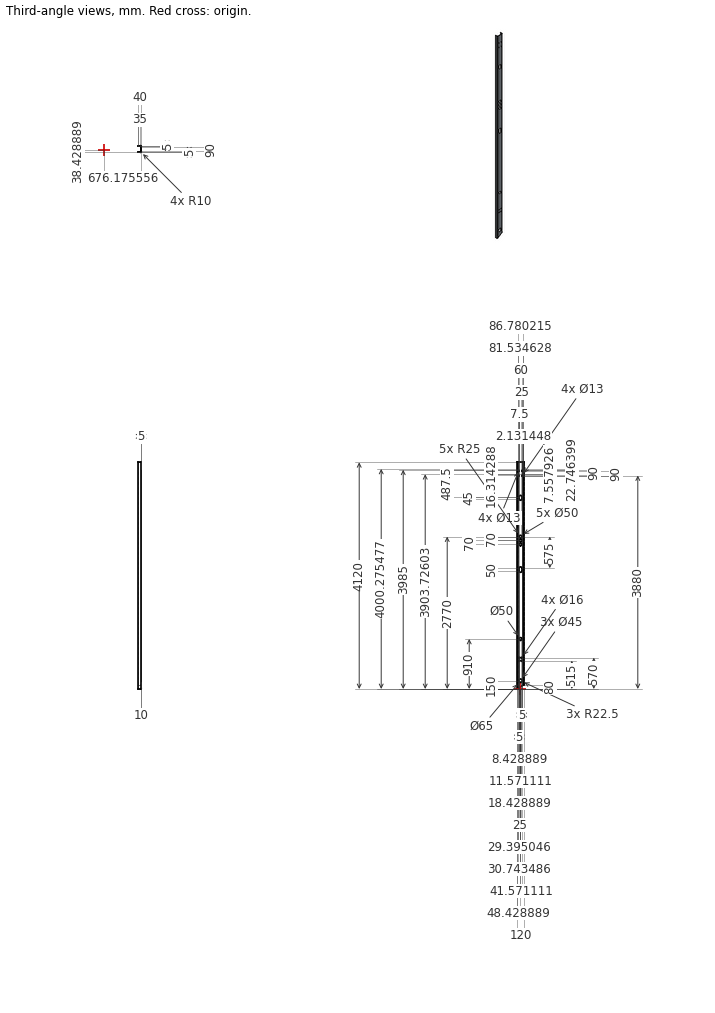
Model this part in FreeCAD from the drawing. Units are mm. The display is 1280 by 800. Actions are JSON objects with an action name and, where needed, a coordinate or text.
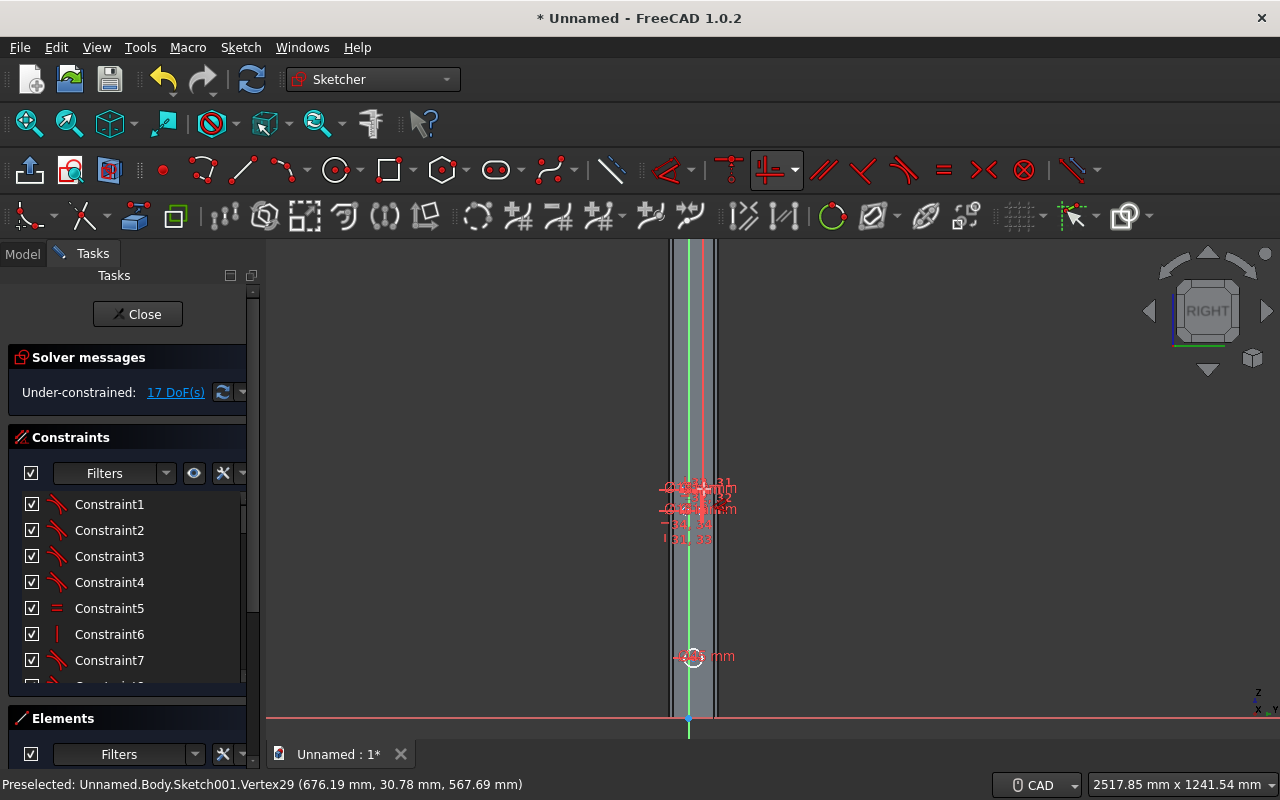
{"action": "scroll", "coordinate": [707, 634], "scroll_direction": "down", "scroll_amount": 8}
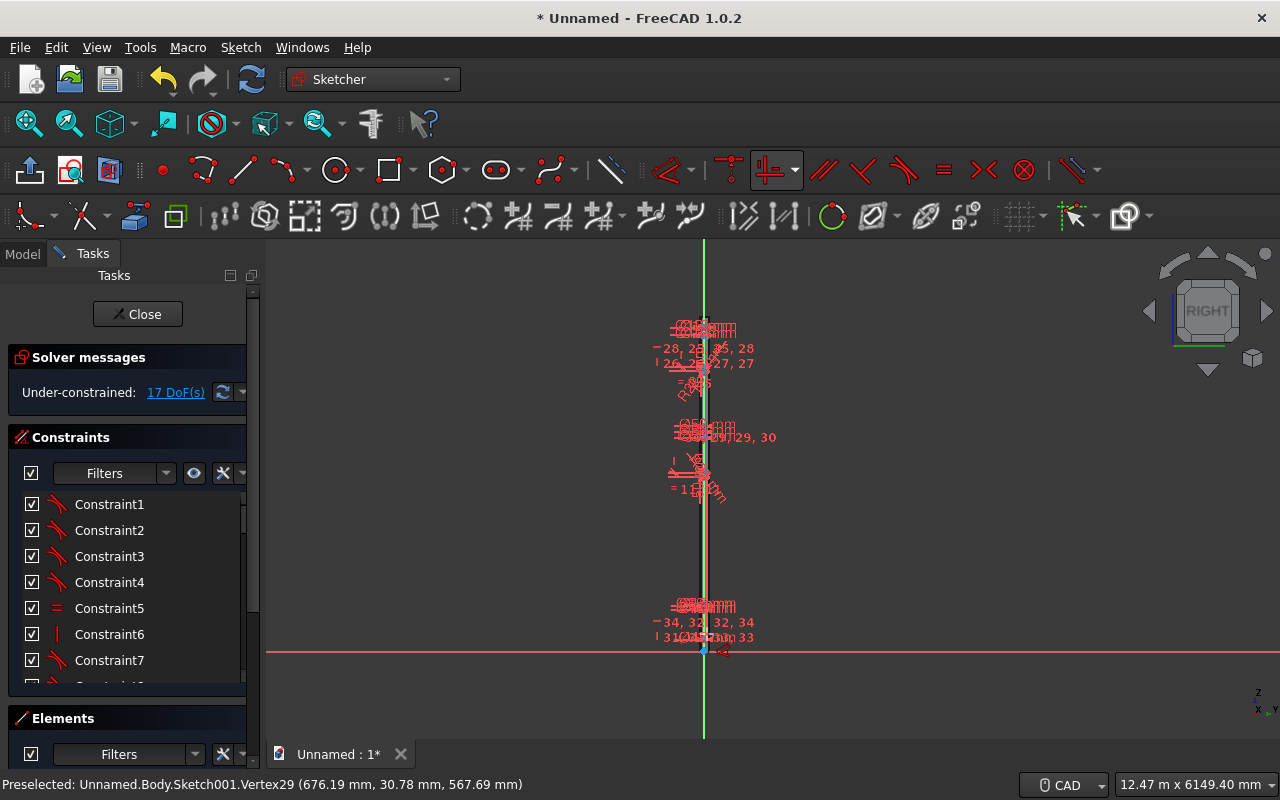
{"action": "scroll", "coordinate": [703, 477], "scroll_direction": "up", "scroll_amount": 23}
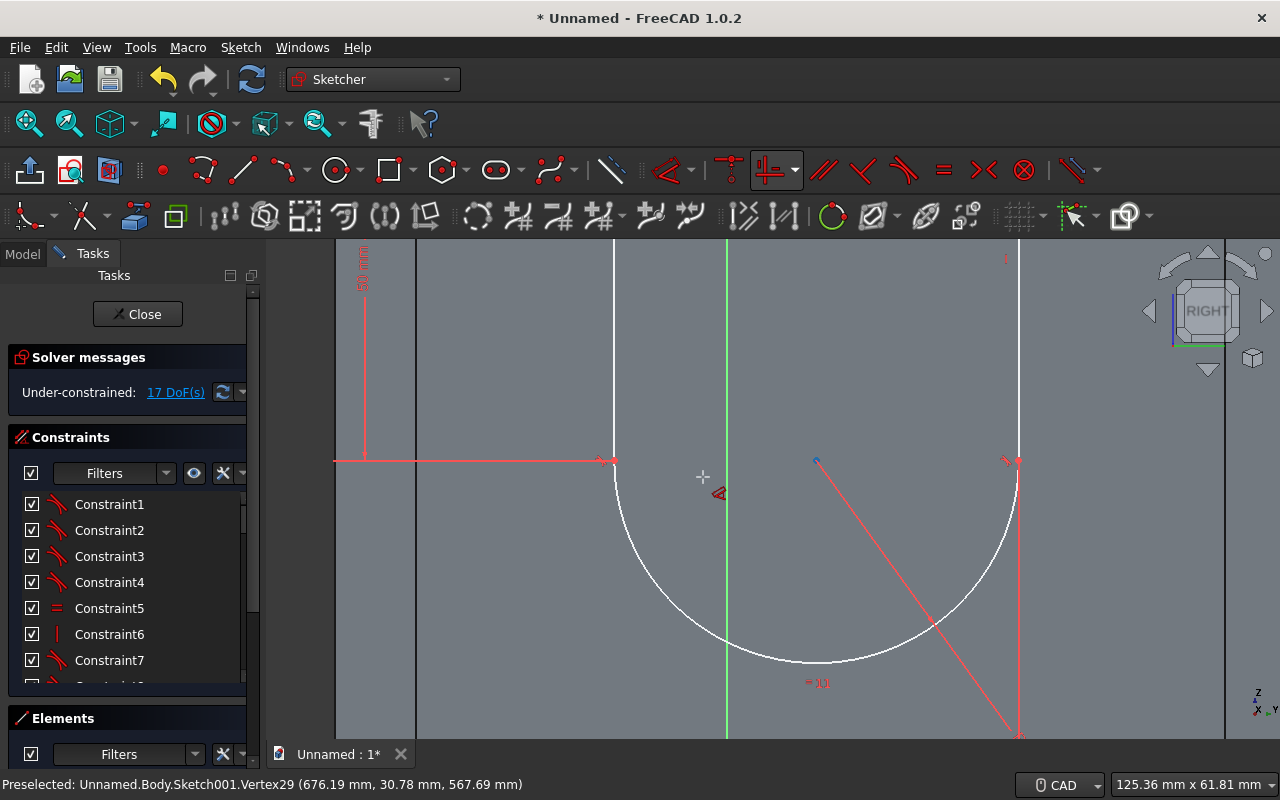
{"action": "left_click", "coordinate": [614, 461]}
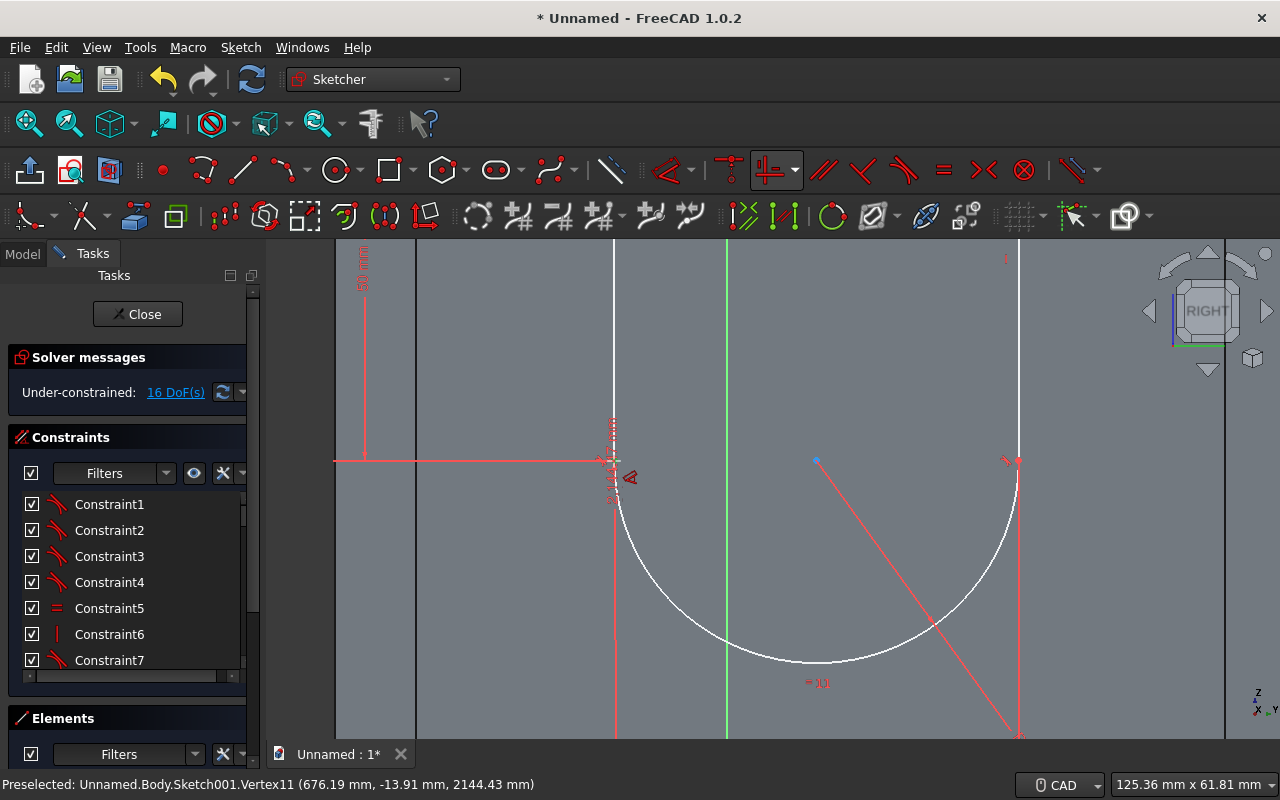
{"action": "scroll", "coordinate": [704, 489], "scroll_direction": "down", "scroll_amount": 15}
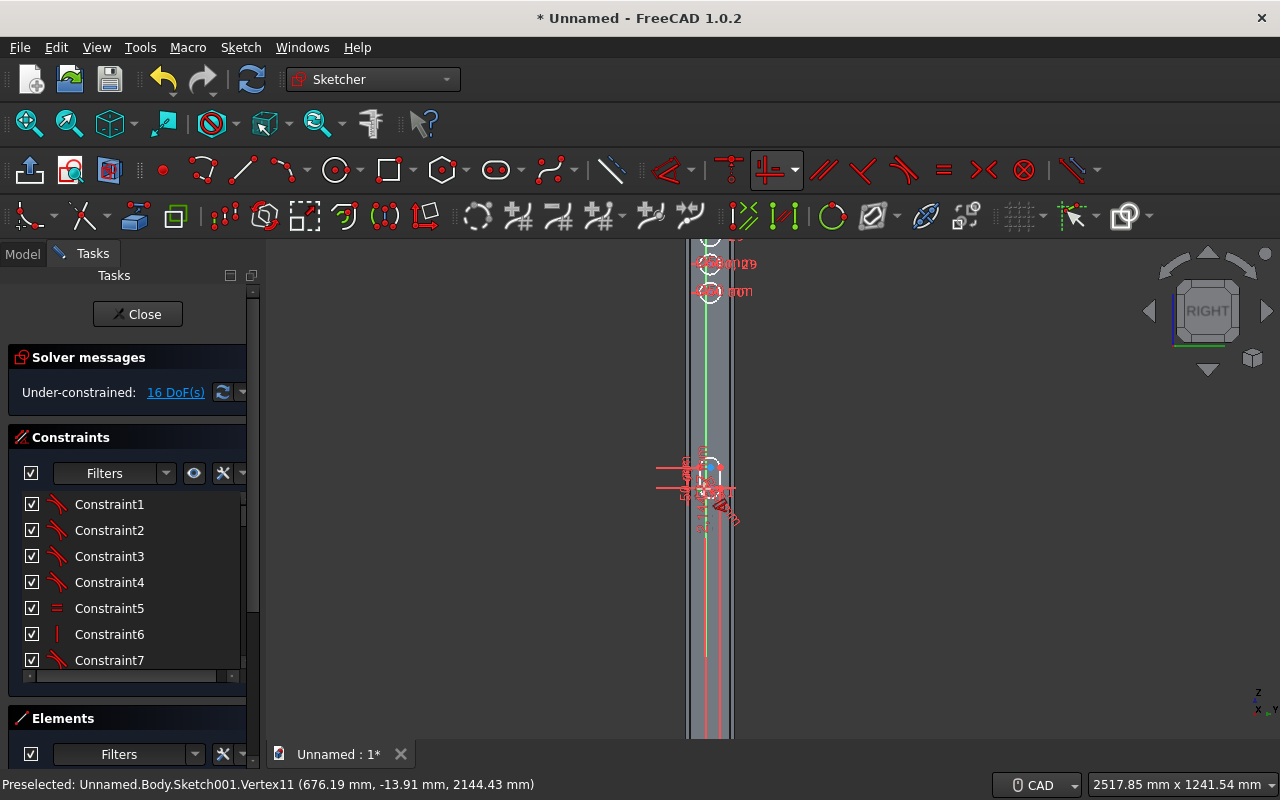
{"action": "scroll", "coordinate": [703, 474], "scroll_direction": "down", "scroll_amount": 8}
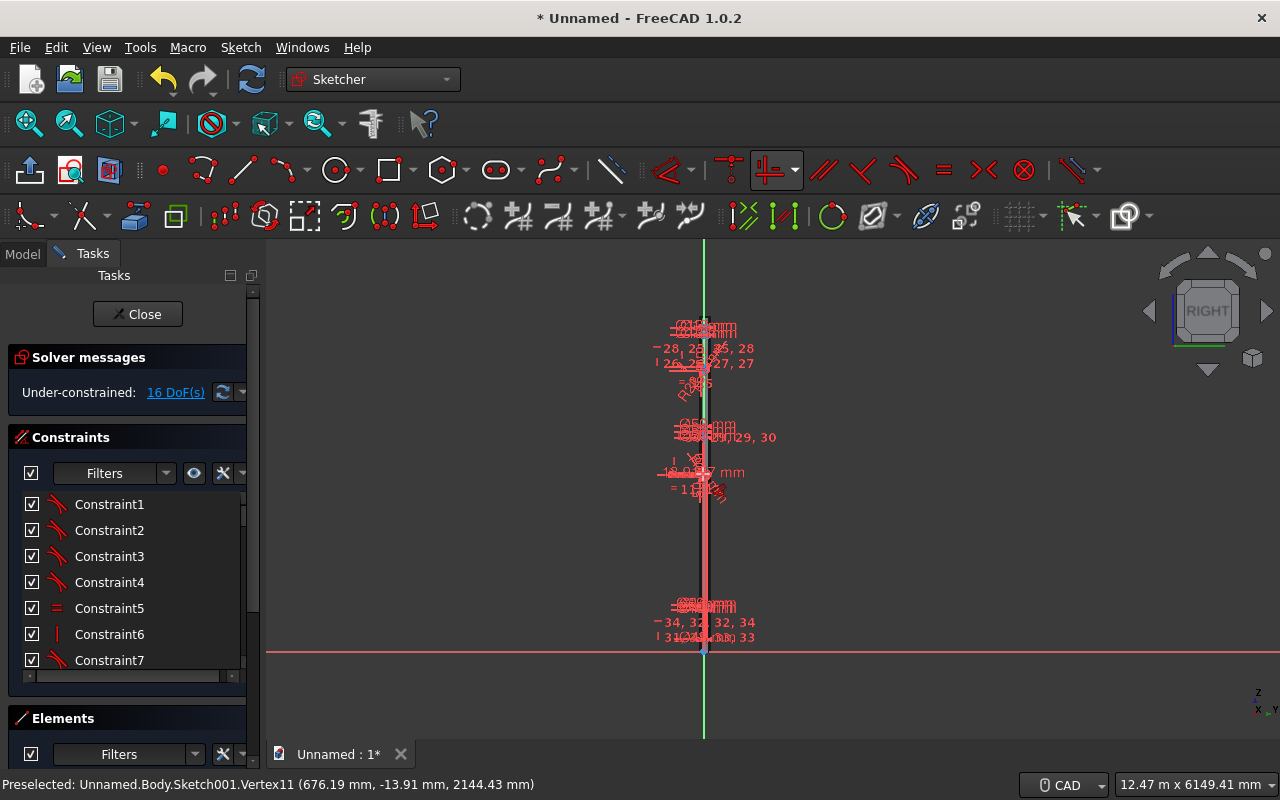
{"action": "scroll", "coordinate": [703, 605], "scroll_direction": "up", "scroll_amount": 23}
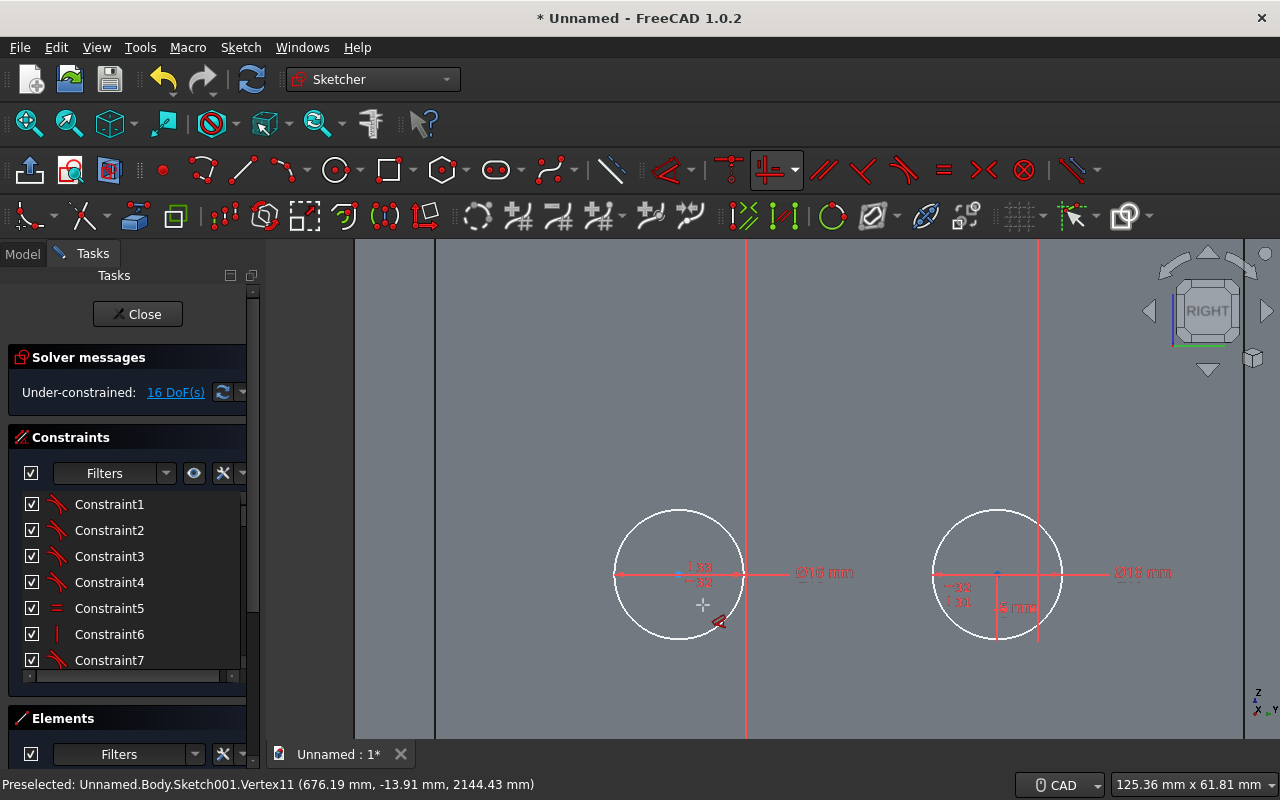
{"action": "left_click", "coordinate": [679, 575]}
{"action": "left_click", "coordinate": [656, 609]}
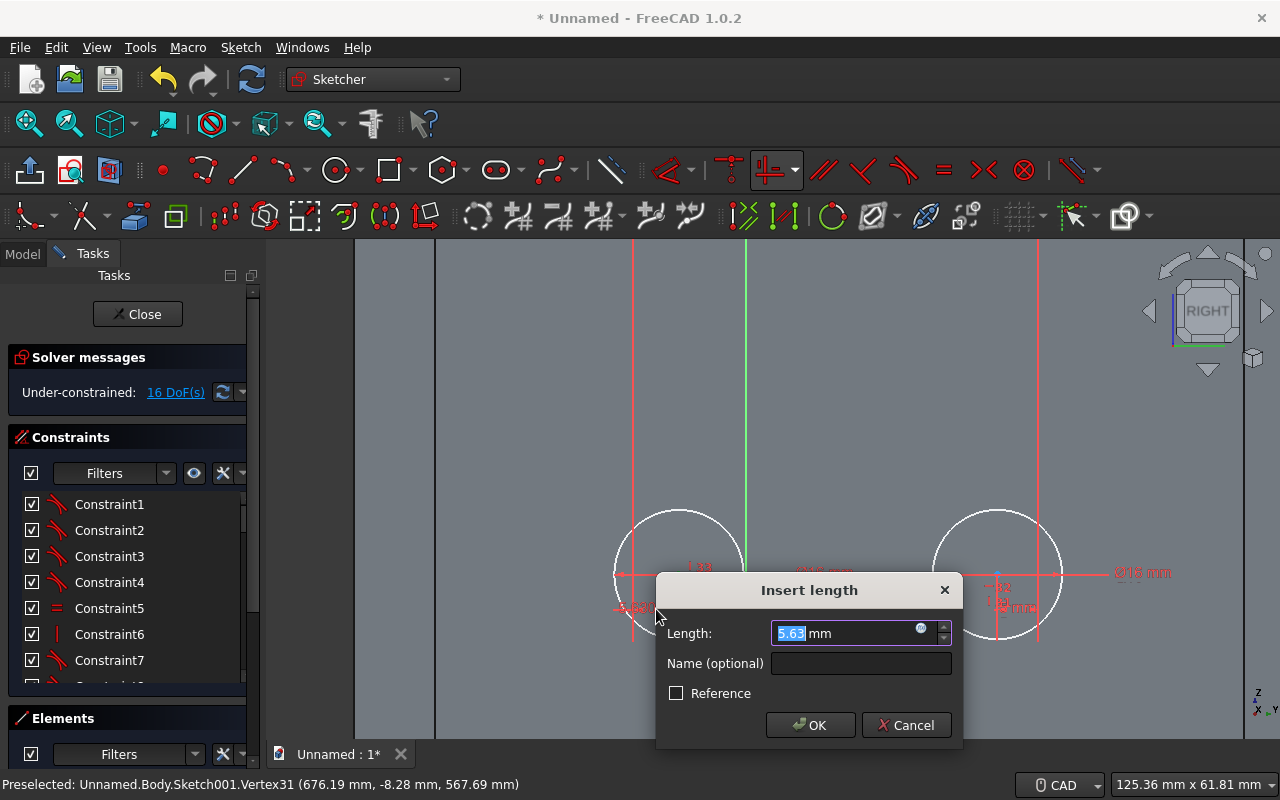
{"action": "type", "text": "5"}
{"action": "key", "text": "Return"}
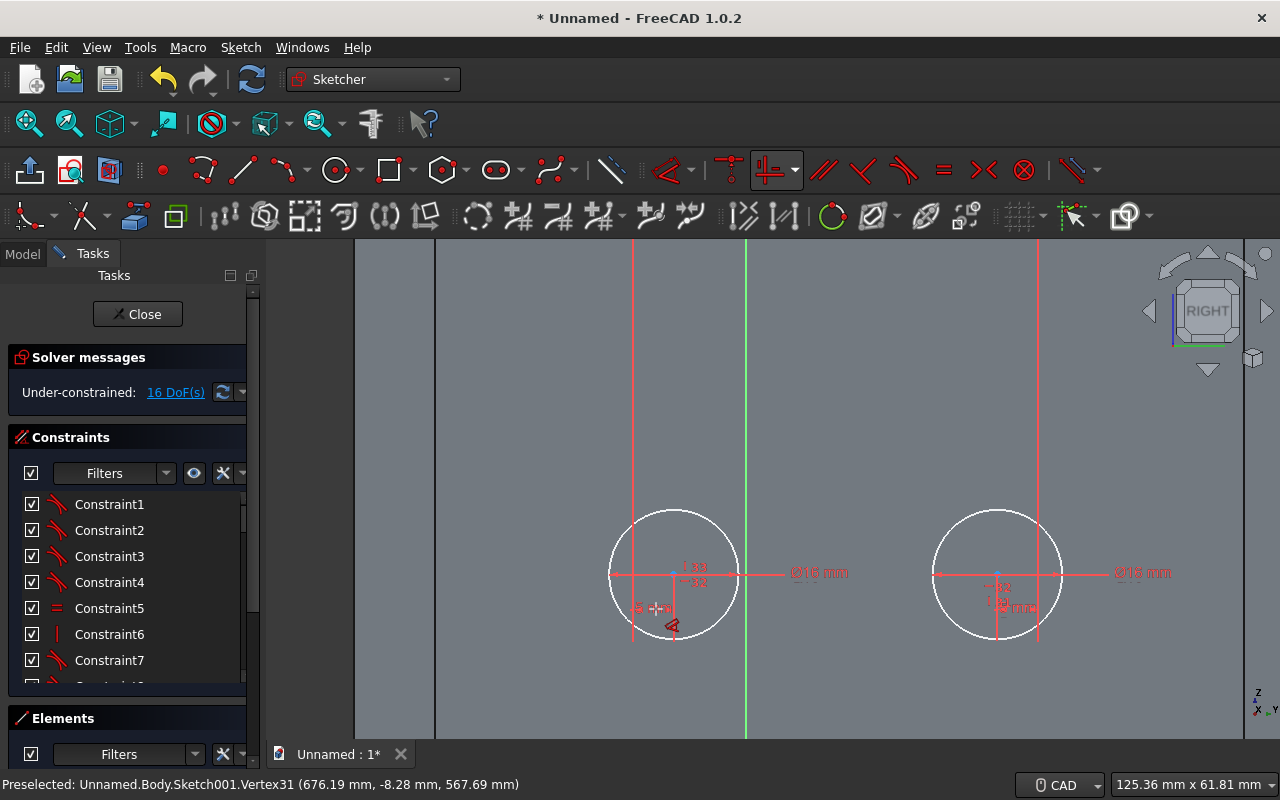
{"action": "scroll", "coordinate": [704, 489], "scroll_direction": "down", "scroll_amount": 15}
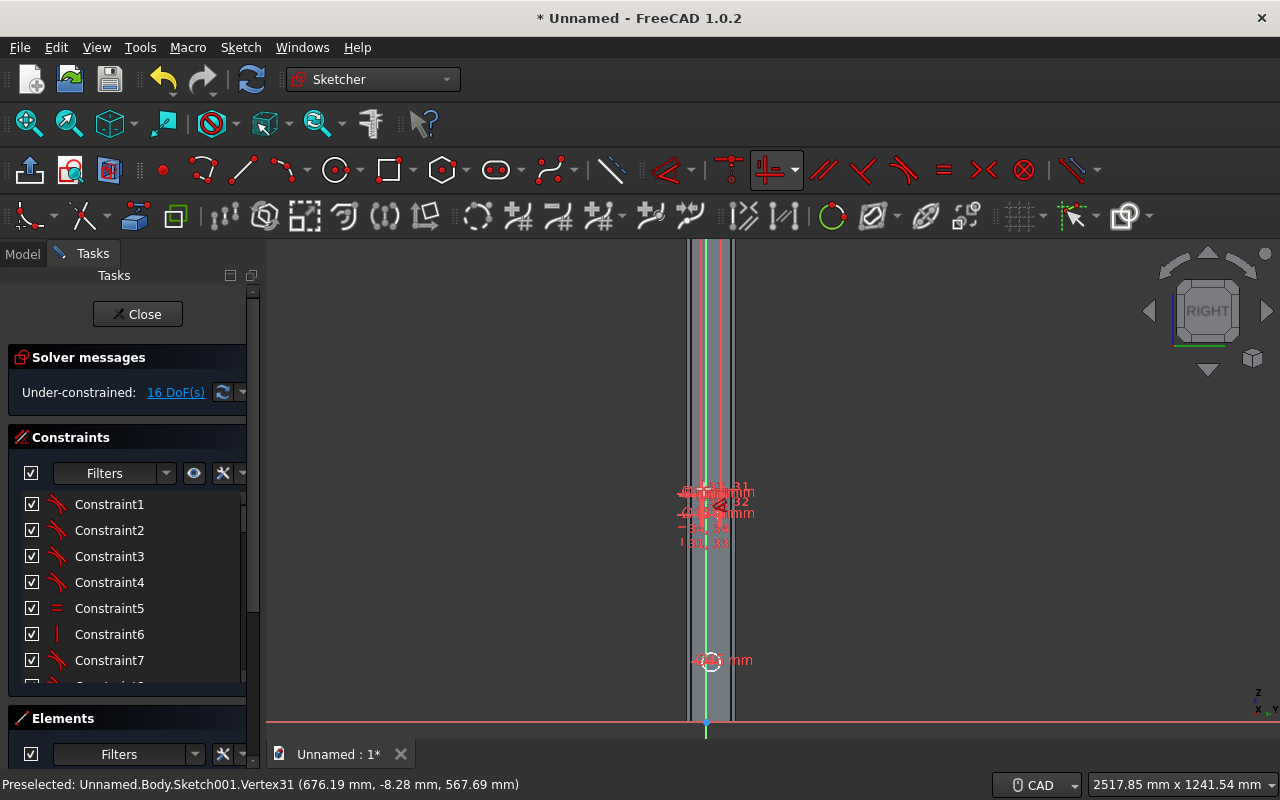
{"action": "scroll", "coordinate": [703, 633], "scroll_direction": "down", "scroll_amount": 8}